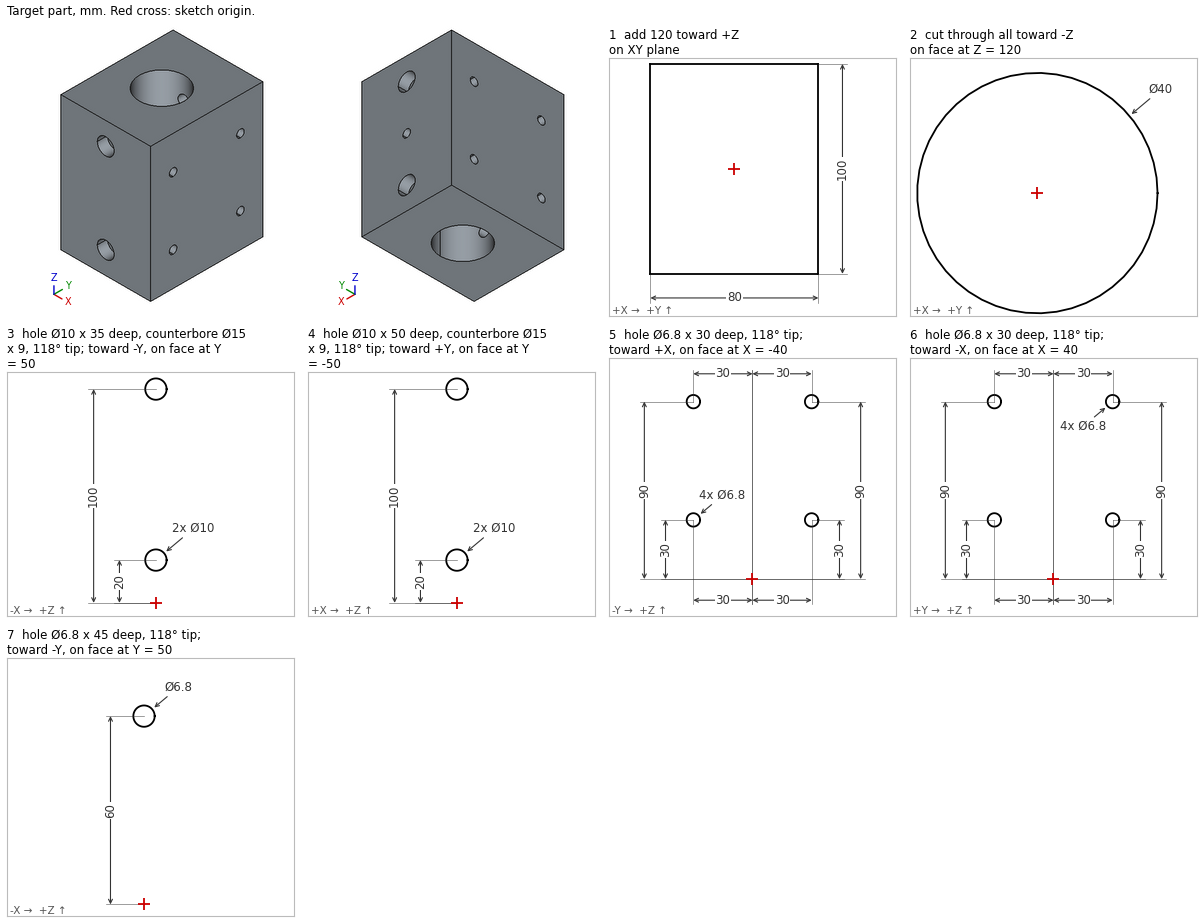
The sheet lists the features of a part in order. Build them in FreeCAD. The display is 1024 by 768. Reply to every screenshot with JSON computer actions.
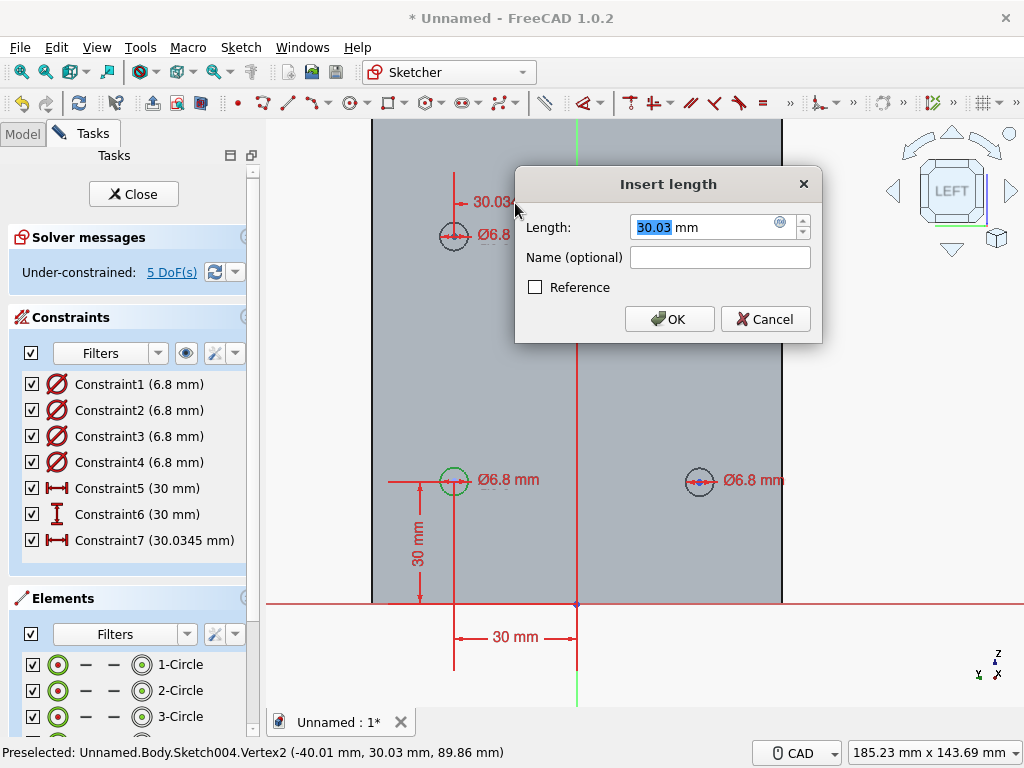
{"action": "type", "text": "30"}
{"action": "key", "text": "Return"}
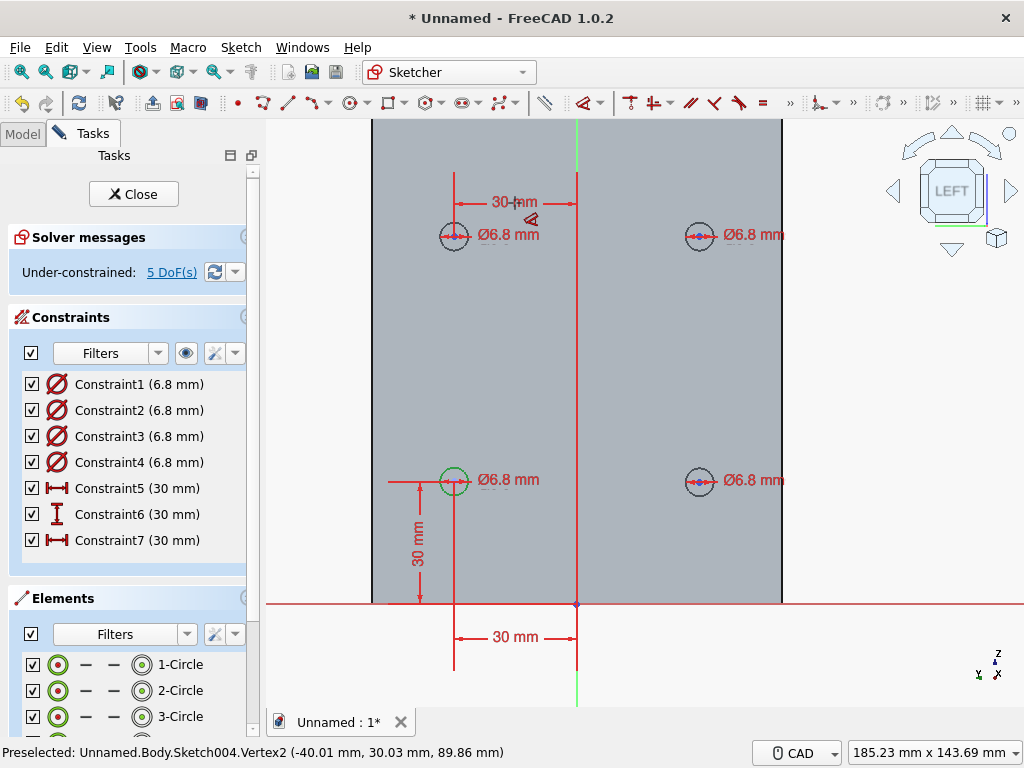
{"action": "left_click", "coordinate": [454, 237]}
{"action": "left_click", "coordinate": [420, 421]}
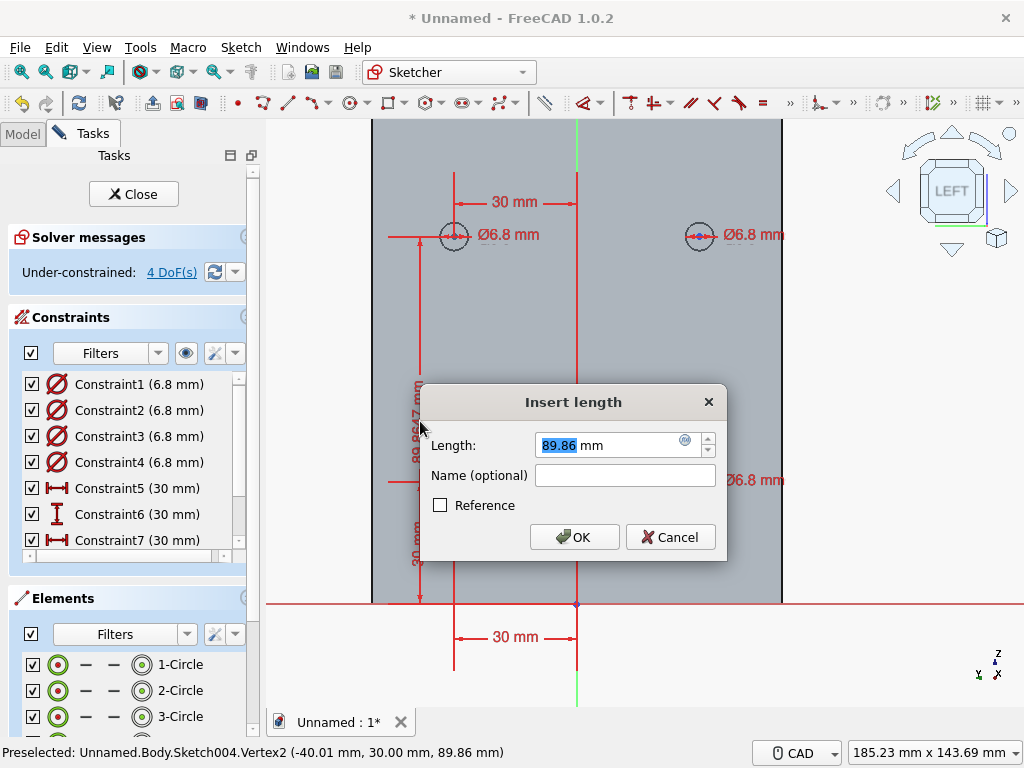
{"action": "type", "text": "90"}
{"action": "key", "text": "Return"}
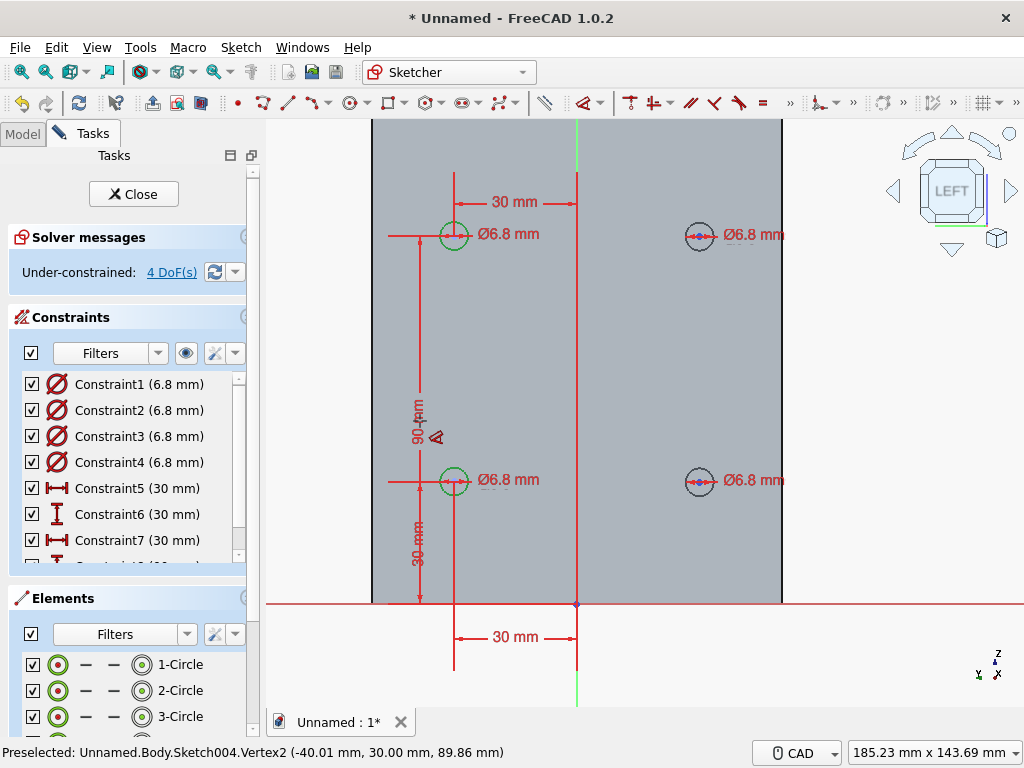
{"action": "left_click", "coordinate": [700, 237]}
{"action": "left_click", "coordinate": [638, 638]}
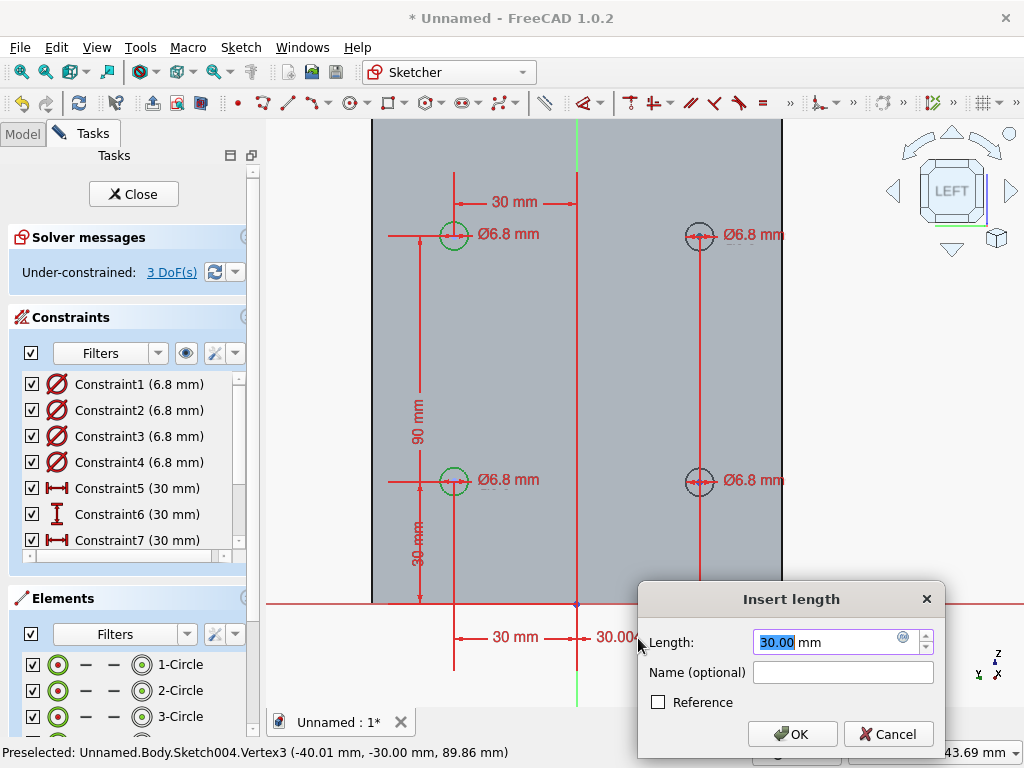
{"action": "type", "text": "30"}
{"action": "key", "text": "Return"}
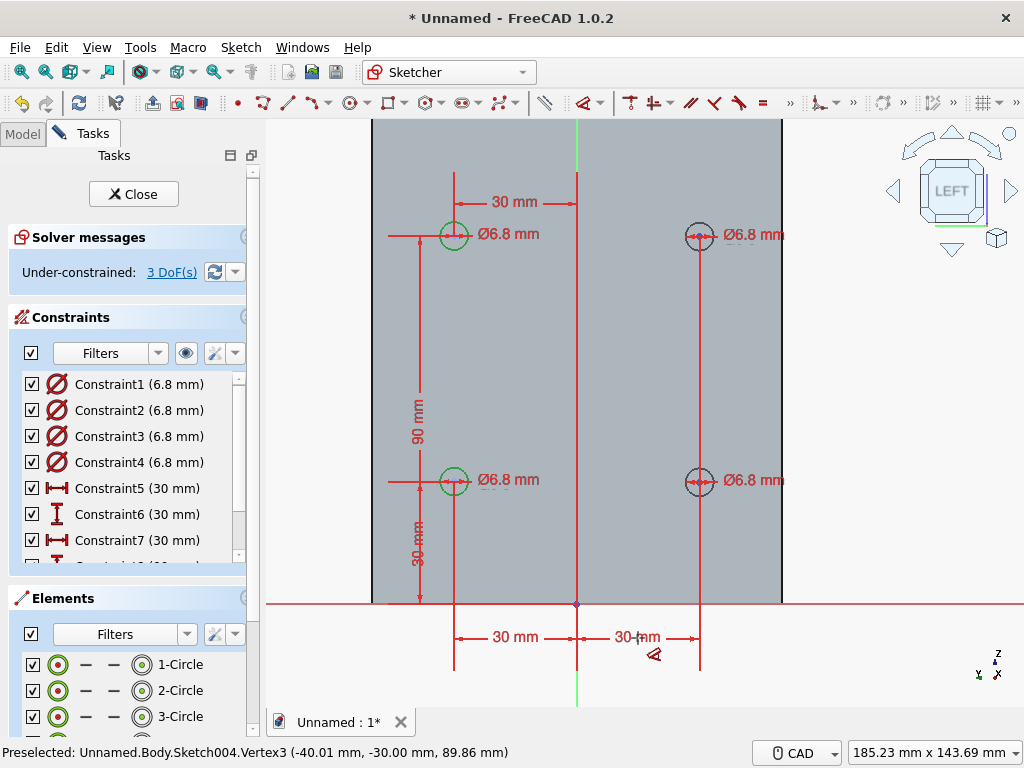
{"action": "left_click", "coordinate": [700, 237]}
{"action": "left_click", "coordinate": [734, 421]}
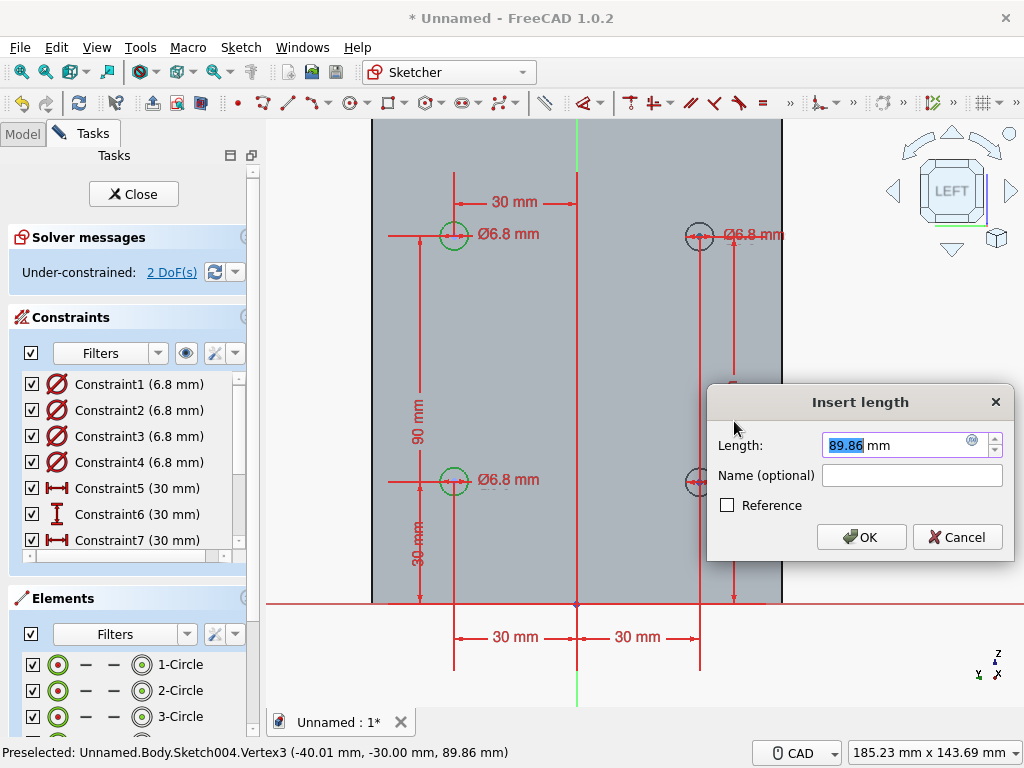
{"action": "type", "text": "90"}
{"action": "key", "text": "Return"}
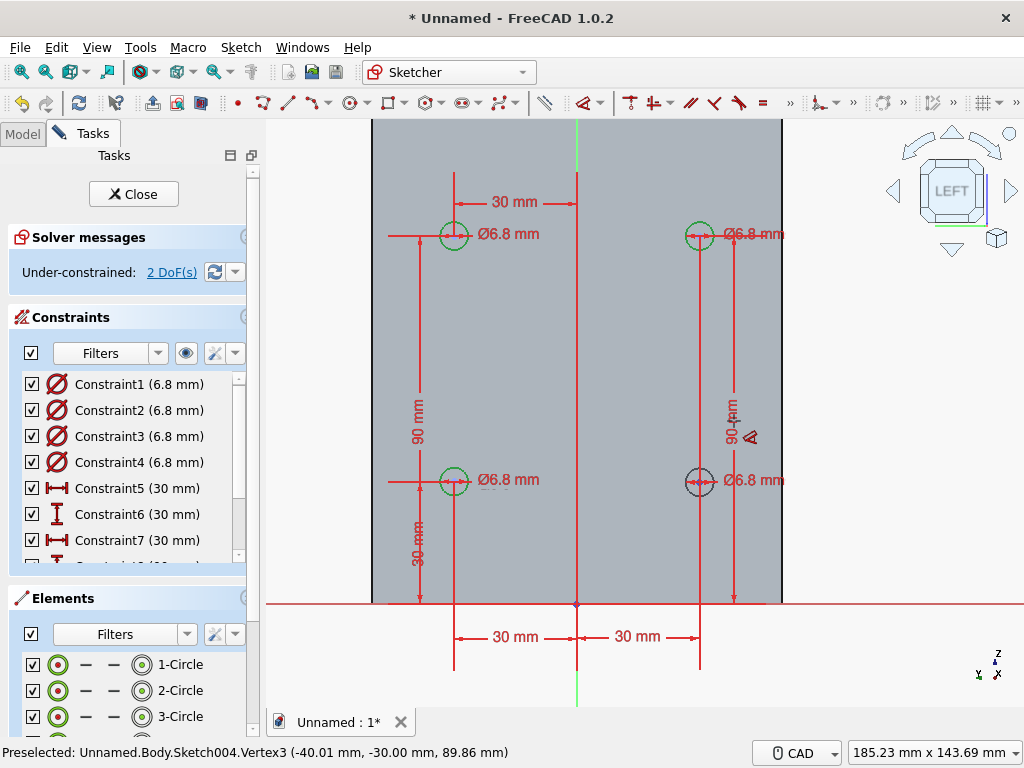
{"action": "left_click", "coordinate": [700, 482]}
{"action": "left_click", "coordinate": [638, 448]}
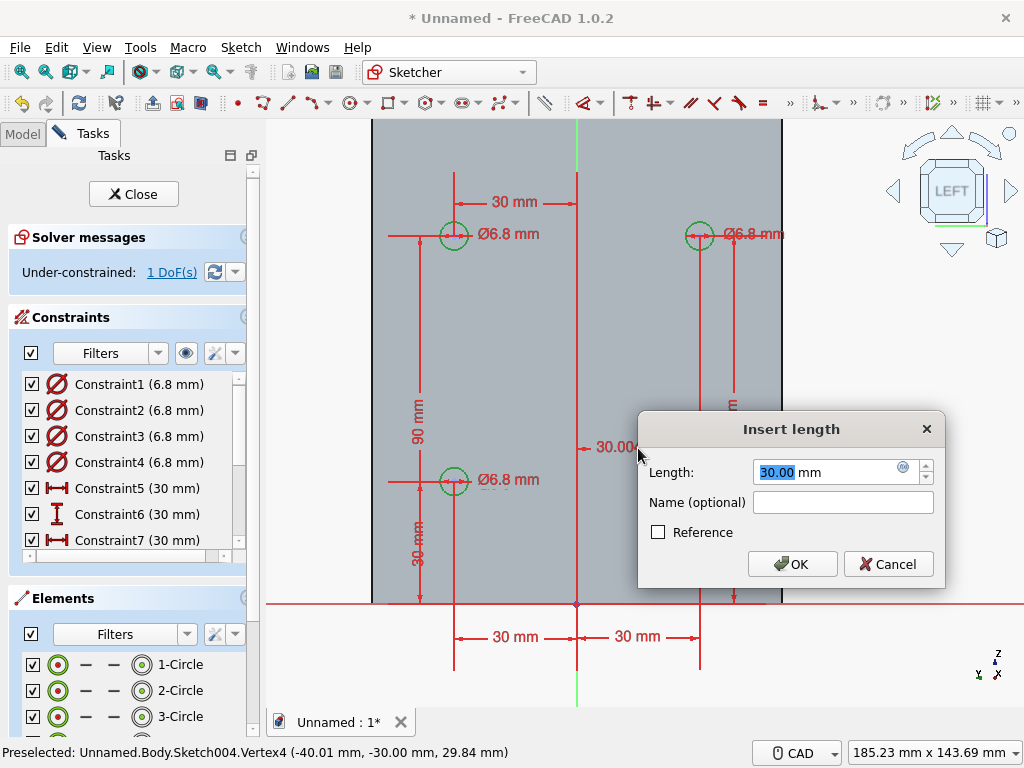
{"action": "type", "text": "30"}
{"action": "key", "text": "Return"}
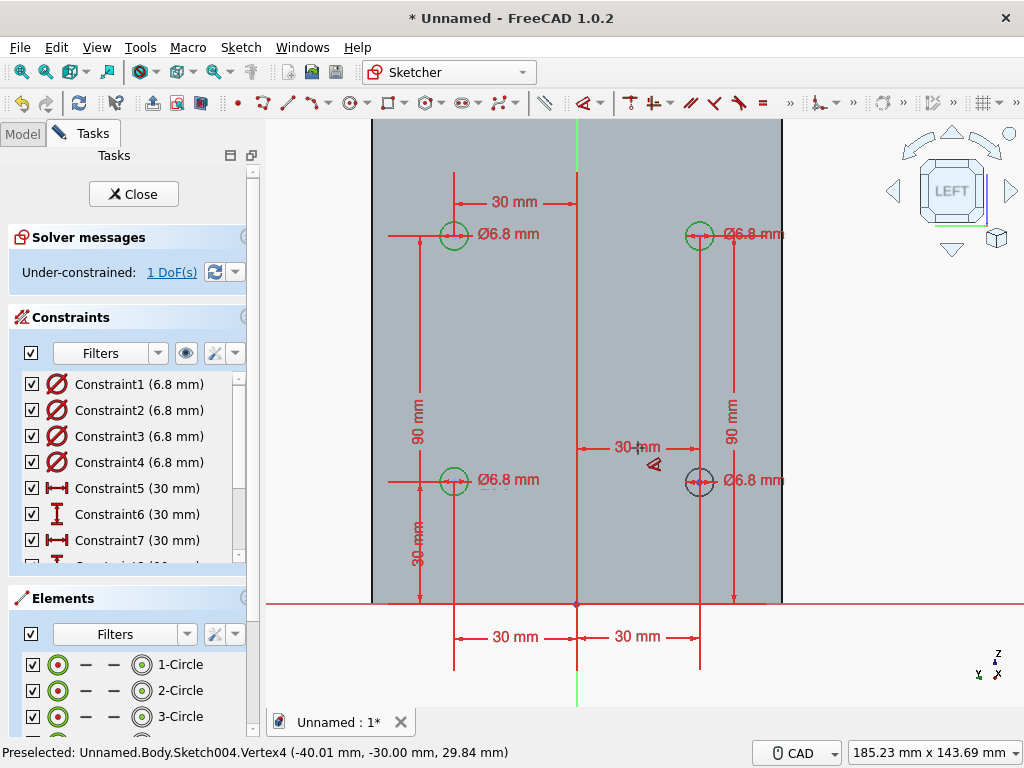
{"action": "left_click", "coordinate": [700, 482]}
{"action": "left_click", "coordinate": [734, 543]}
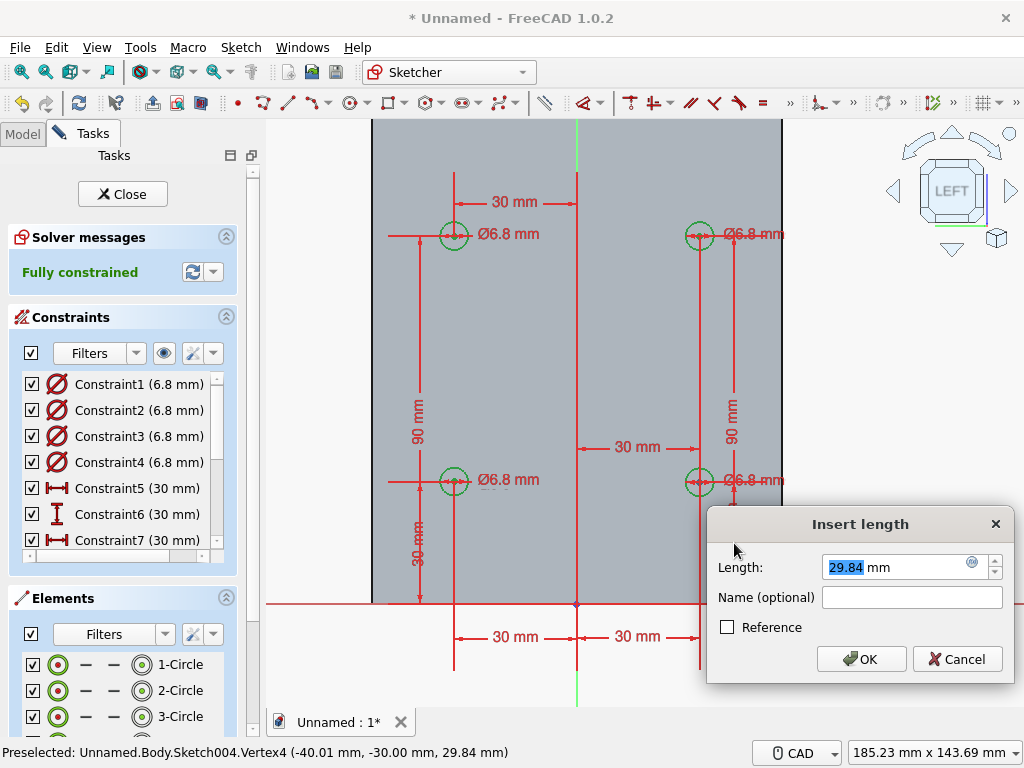
{"action": "type", "text": "30"}
{"action": "key", "text": "Return"}
{"action": "key", "text": "Escape"}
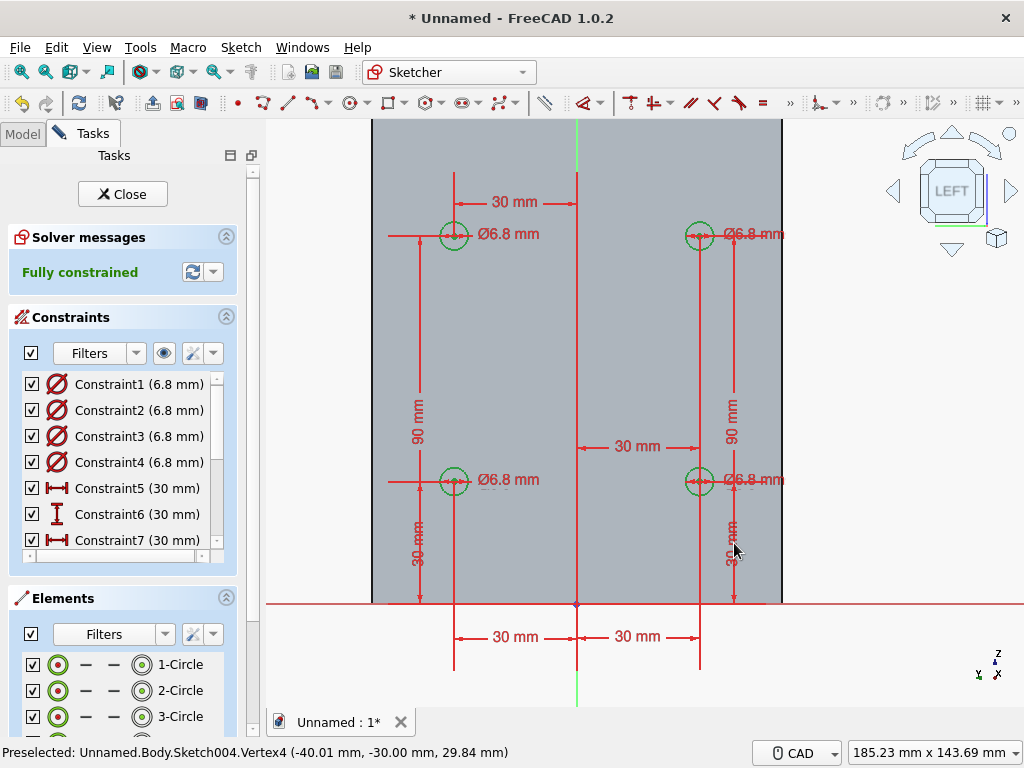
{"action": "left_click", "coordinate": [123, 194]}